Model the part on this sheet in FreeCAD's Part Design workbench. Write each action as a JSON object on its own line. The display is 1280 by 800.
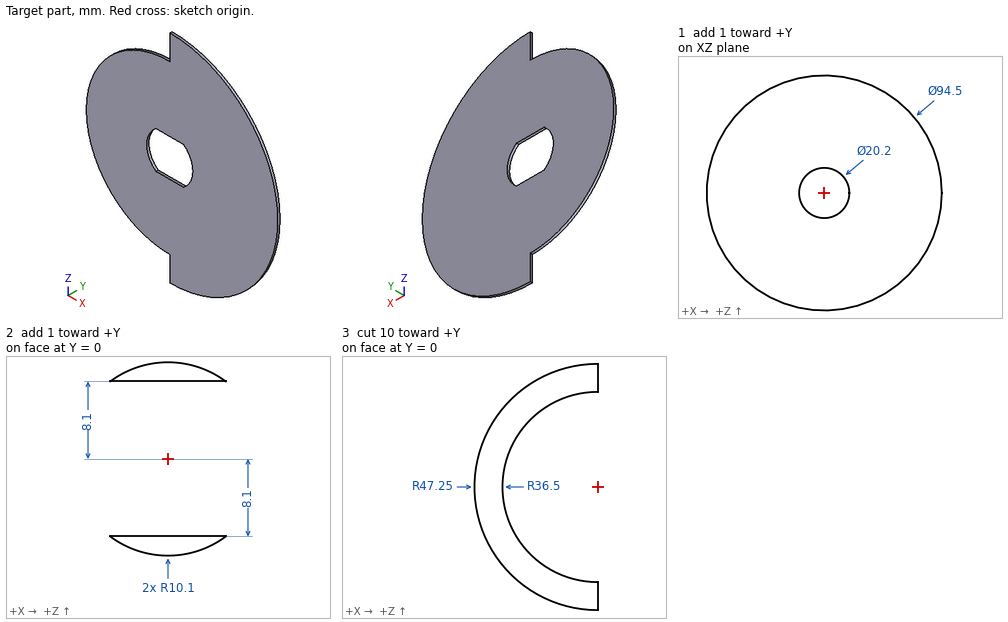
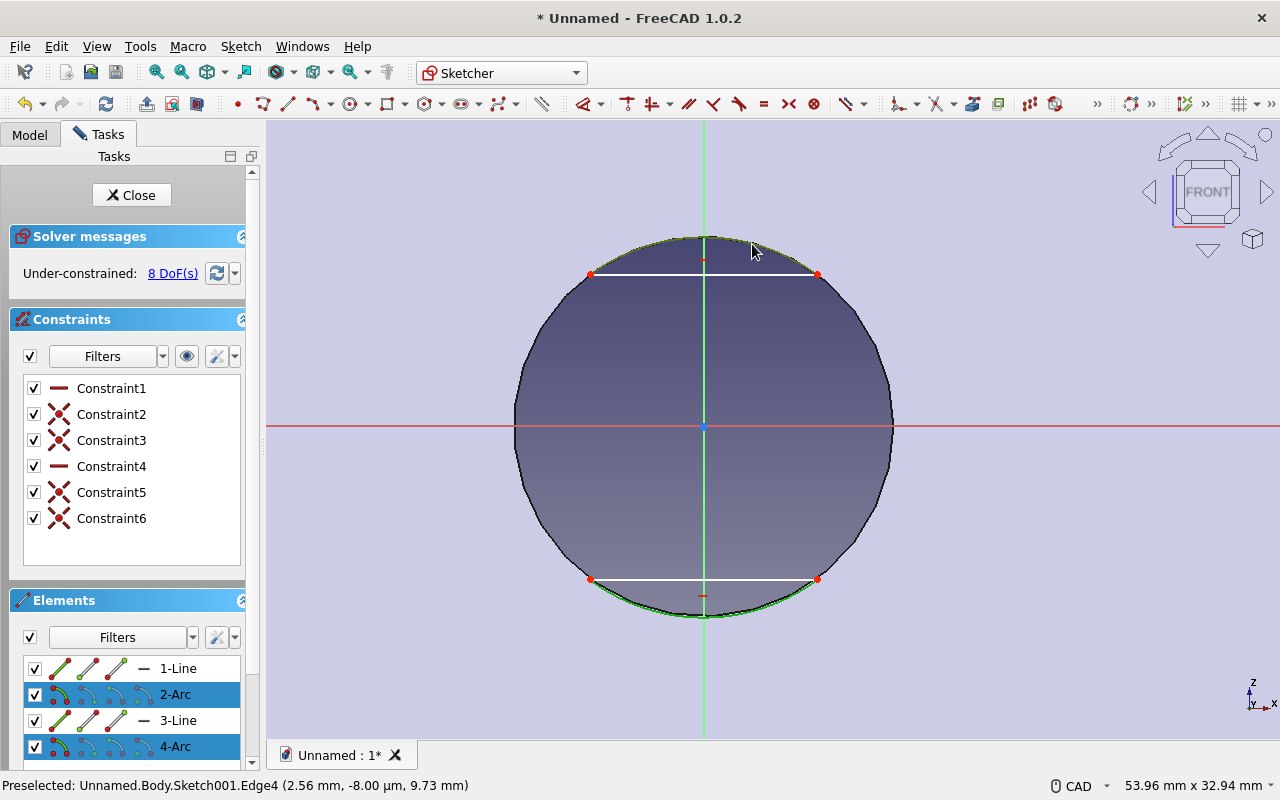
{"action": "left_click", "coordinate": [627, 104]}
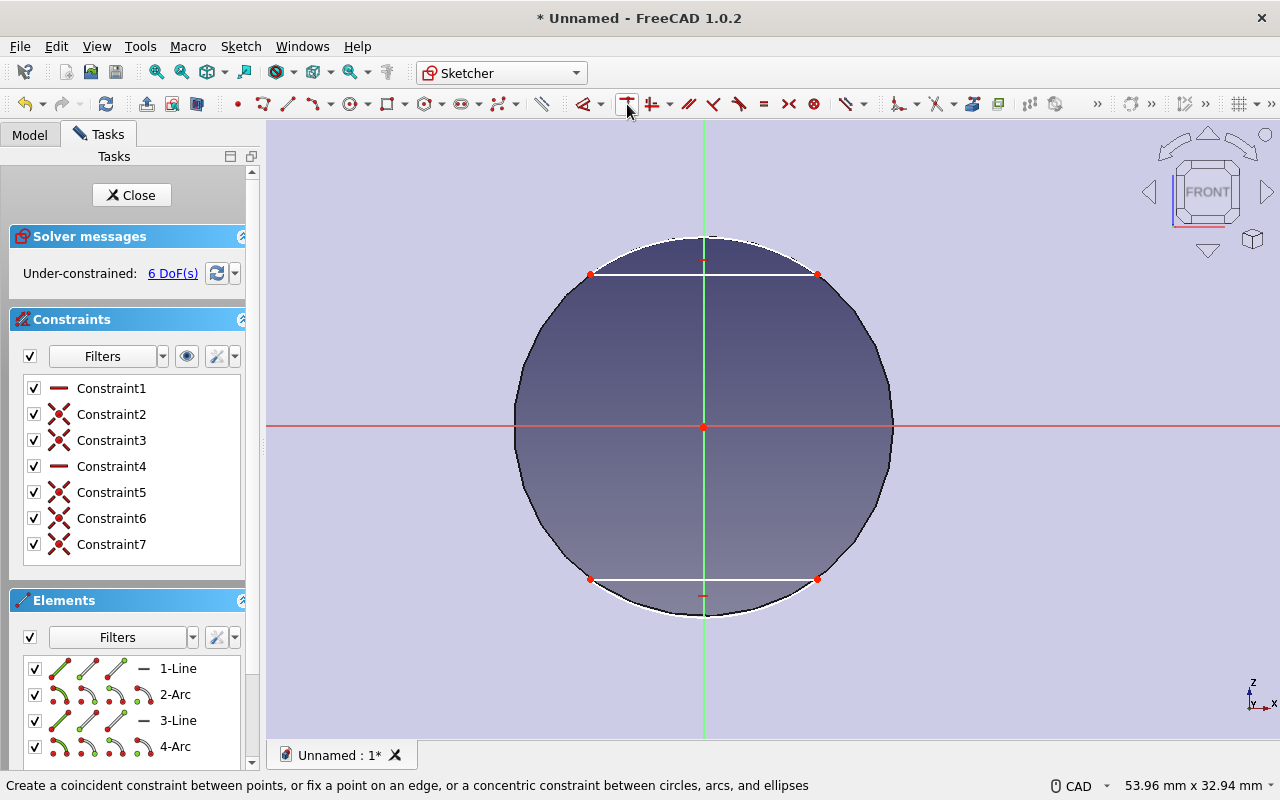
{"action": "left_click_drag", "start_coordinate": [693, 416], "coordinate": [714, 438]}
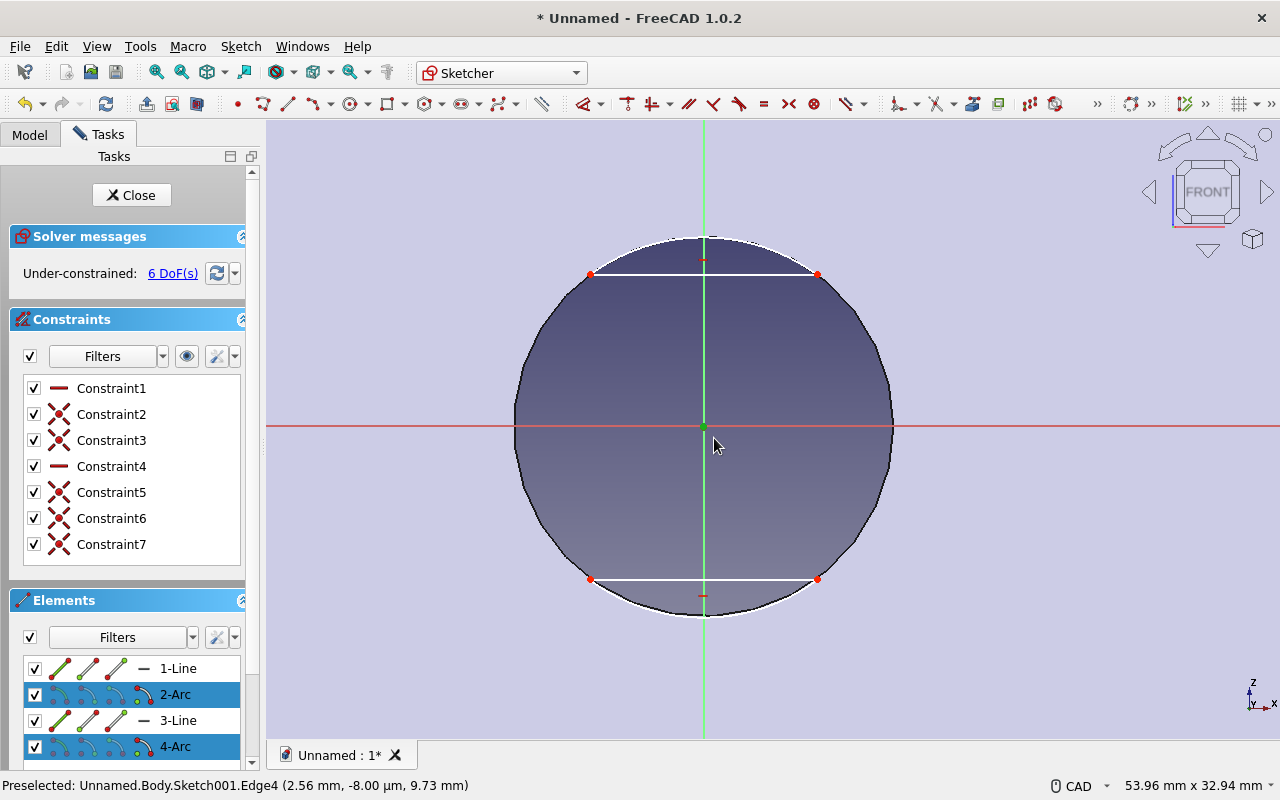
{"action": "left_click", "coordinate": [627, 104]}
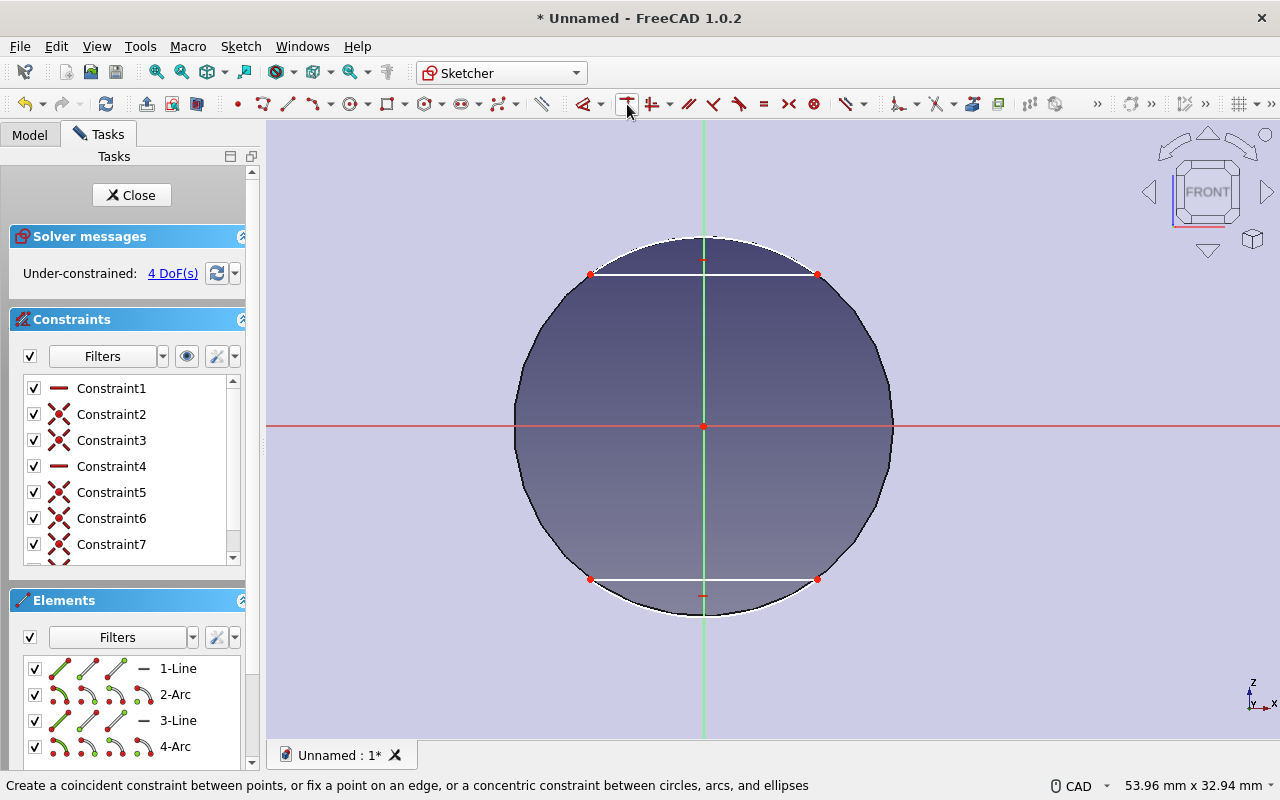
{"action": "left_click", "coordinate": [656, 611]}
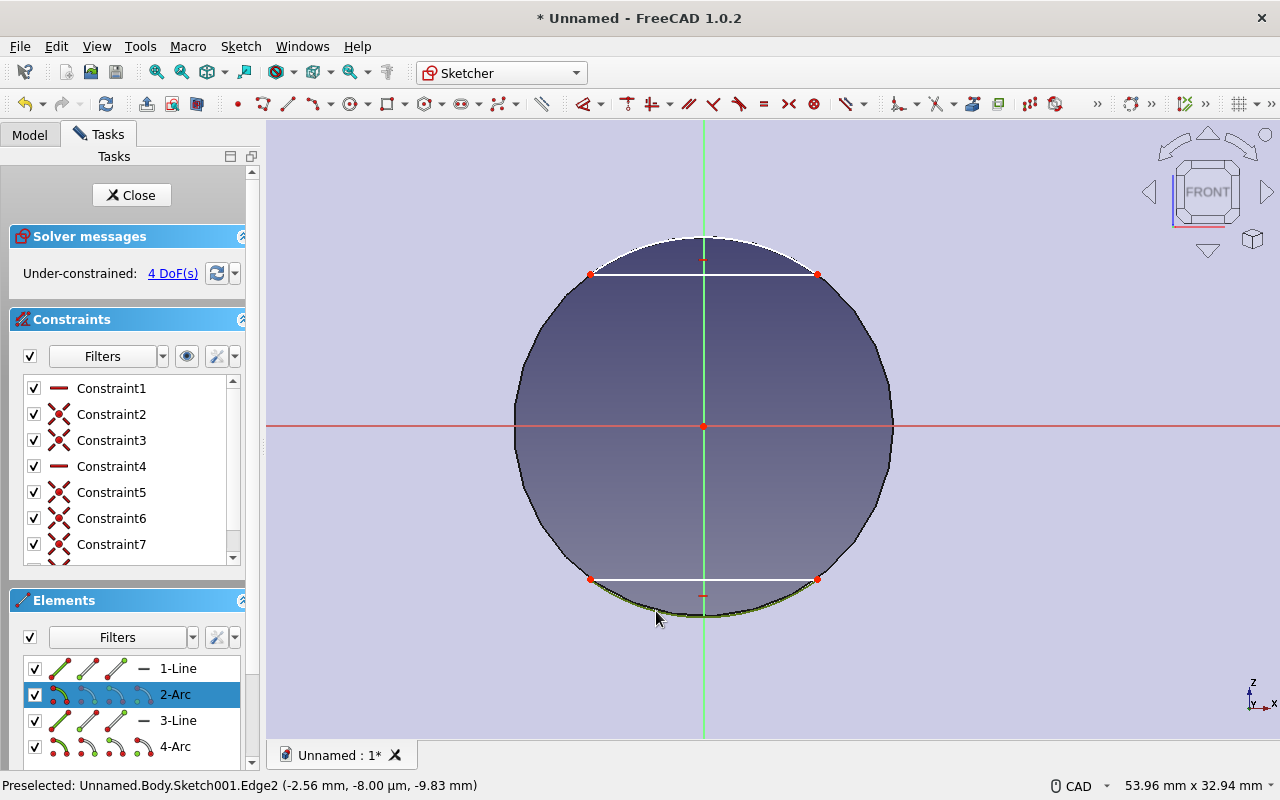
{"action": "left_click", "coordinate": [752, 243]}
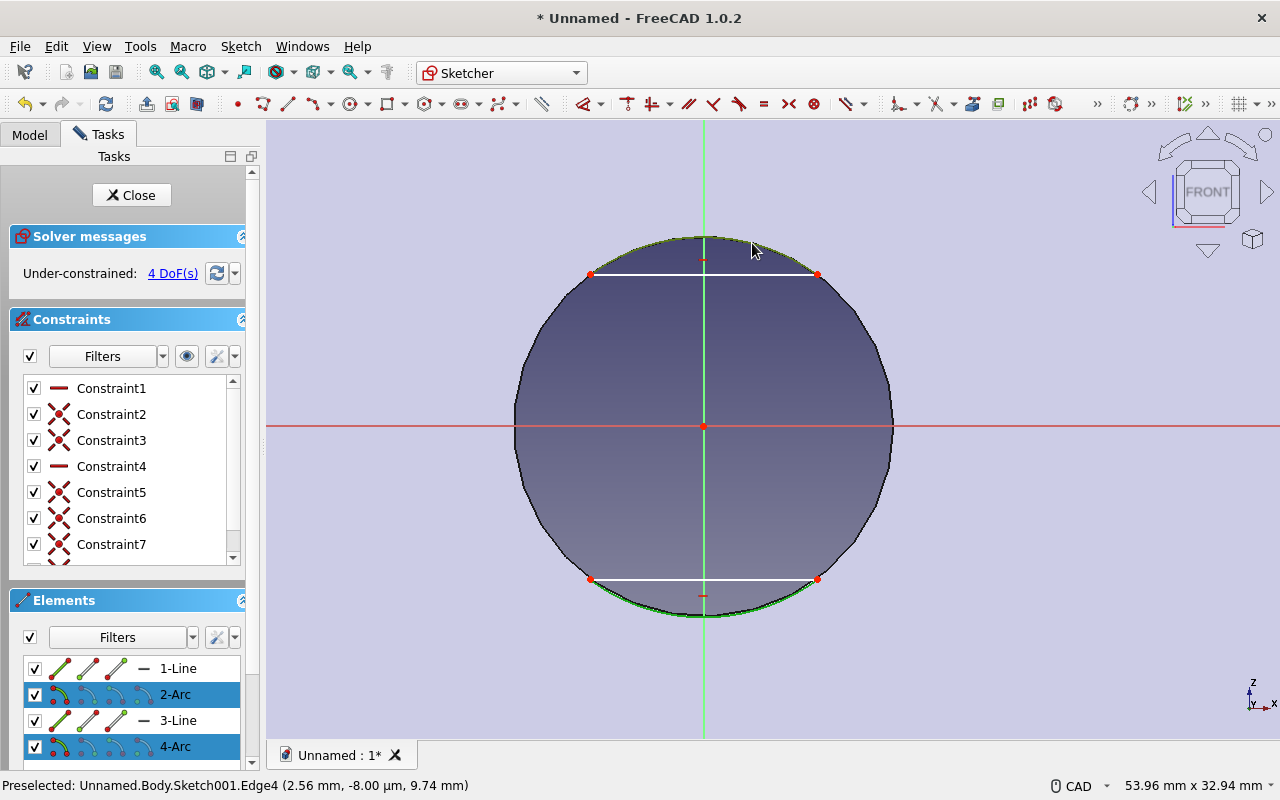
{"action": "left_click", "coordinate": [764, 104]}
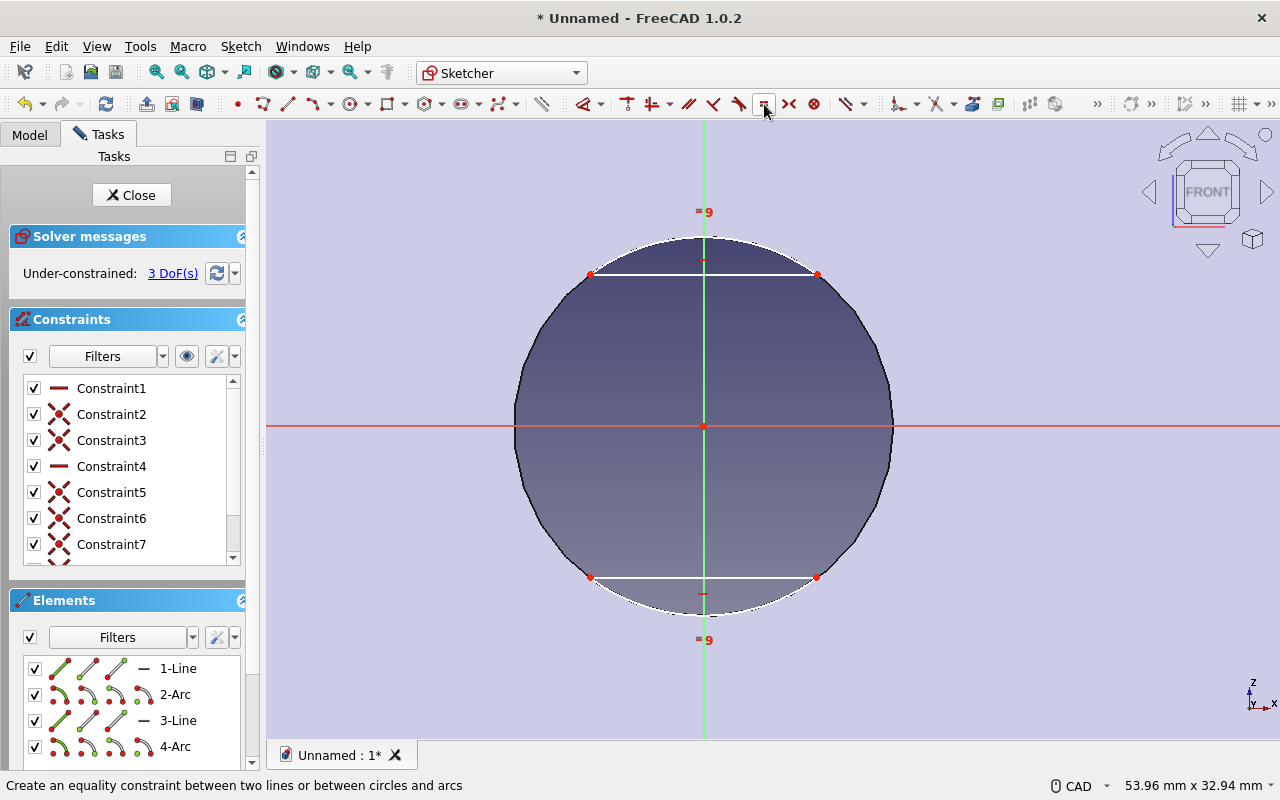
{"action": "left_click", "coordinate": [582, 104]}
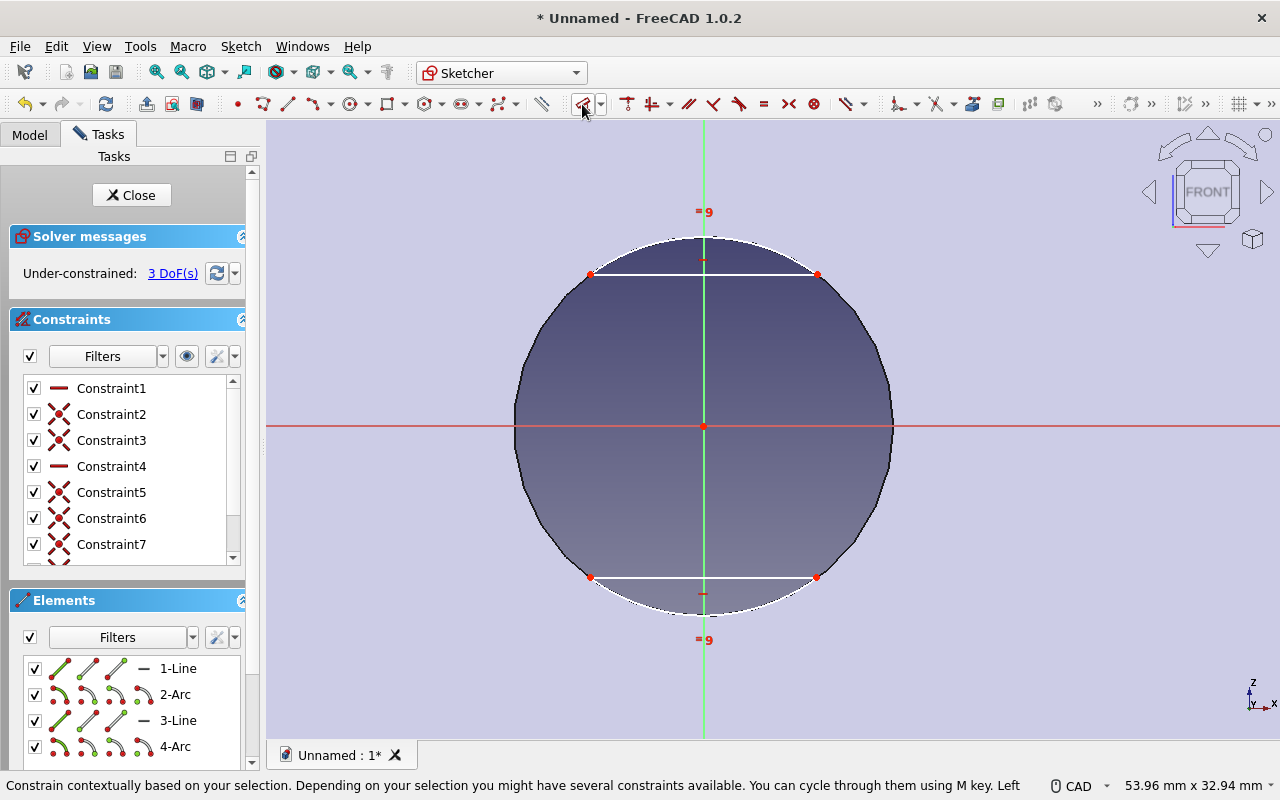
{"action": "left_click", "coordinate": [656, 609]}
{"action": "left_click", "coordinate": [648, 640]}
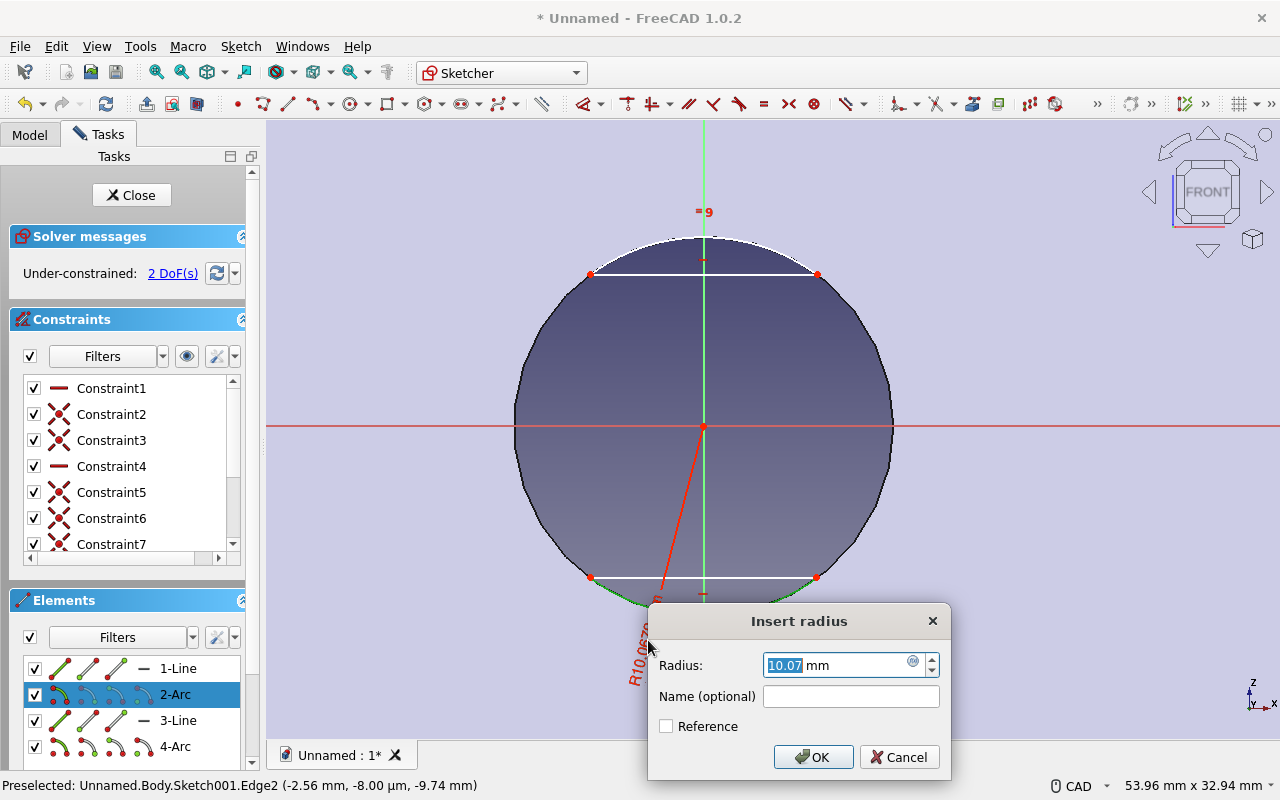
{"action": "type", "text": "10.1"}
{"action": "key", "text": "Return"}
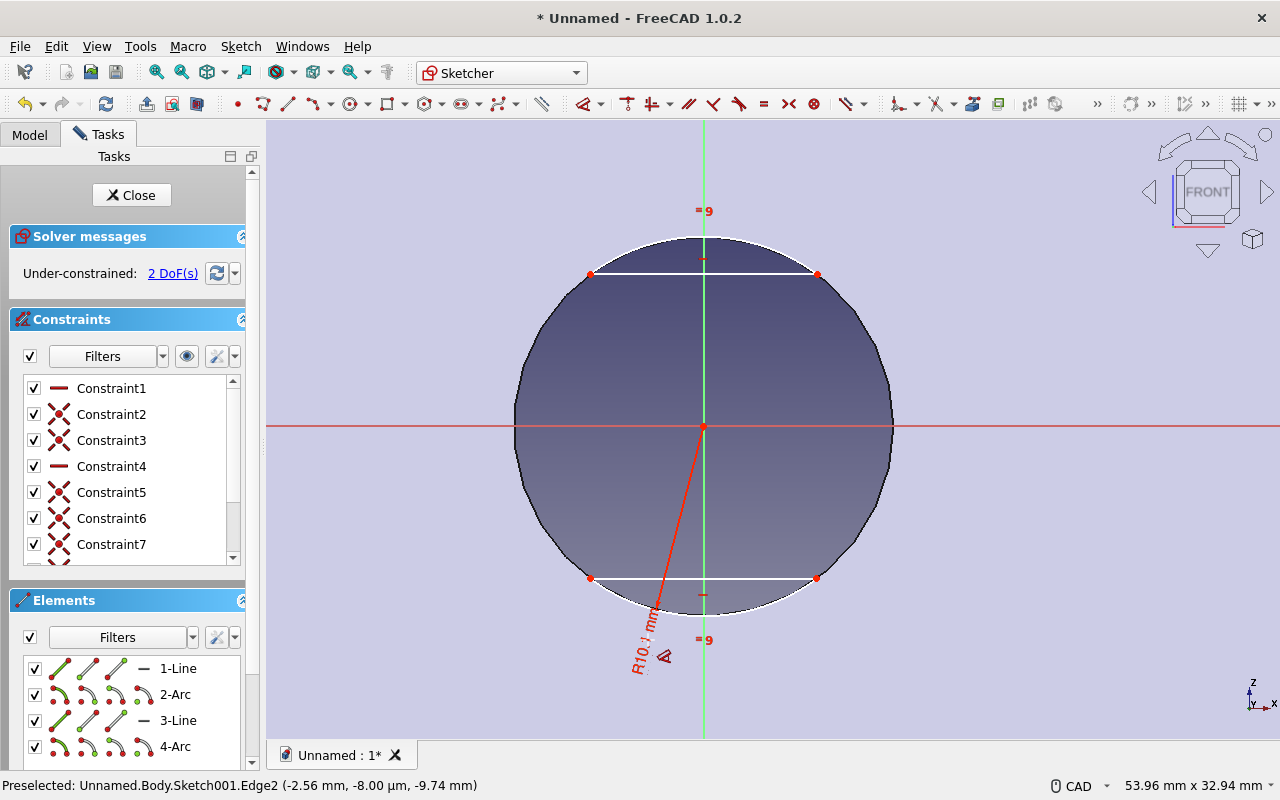
{"action": "left_click", "coordinate": [817, 579]}
{"action": "left_click", "coordinate": [851, 503]}